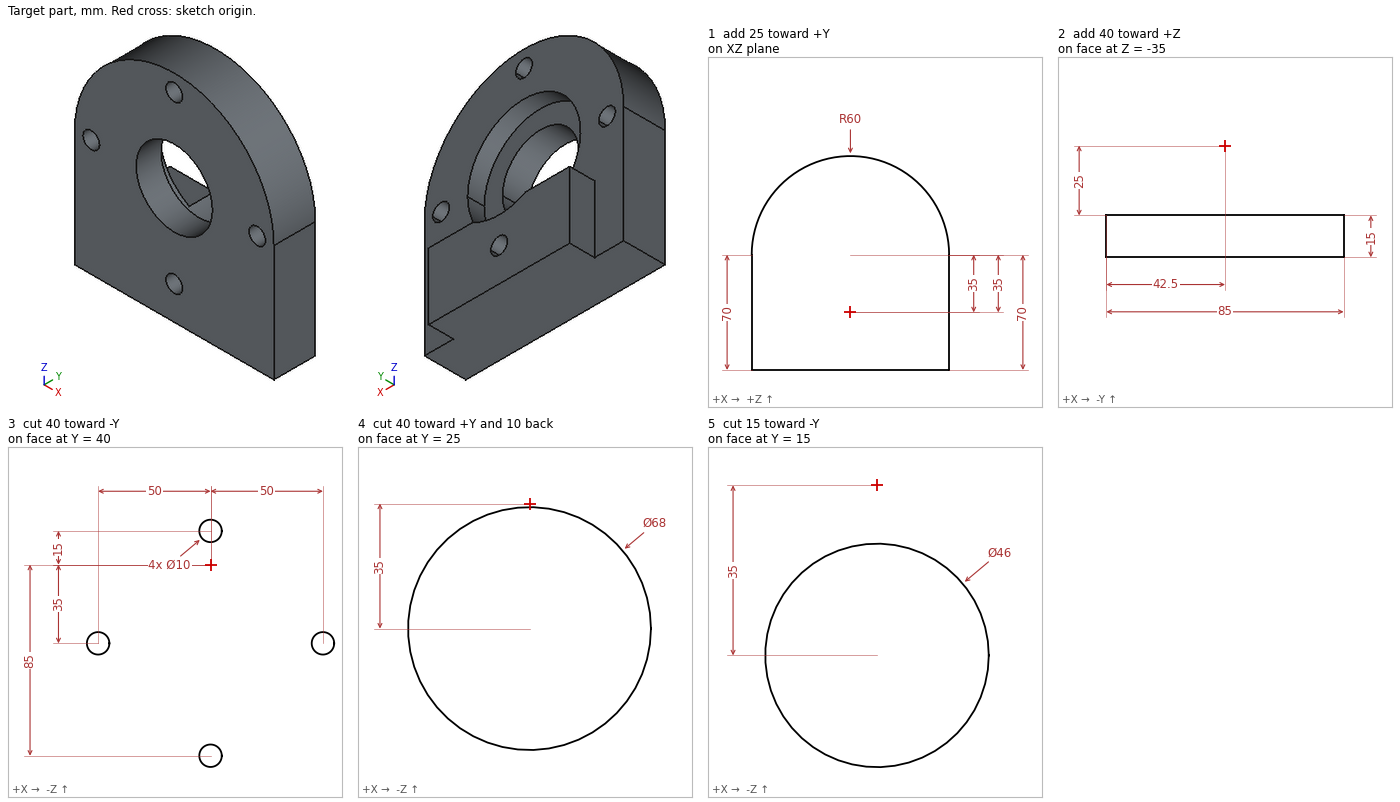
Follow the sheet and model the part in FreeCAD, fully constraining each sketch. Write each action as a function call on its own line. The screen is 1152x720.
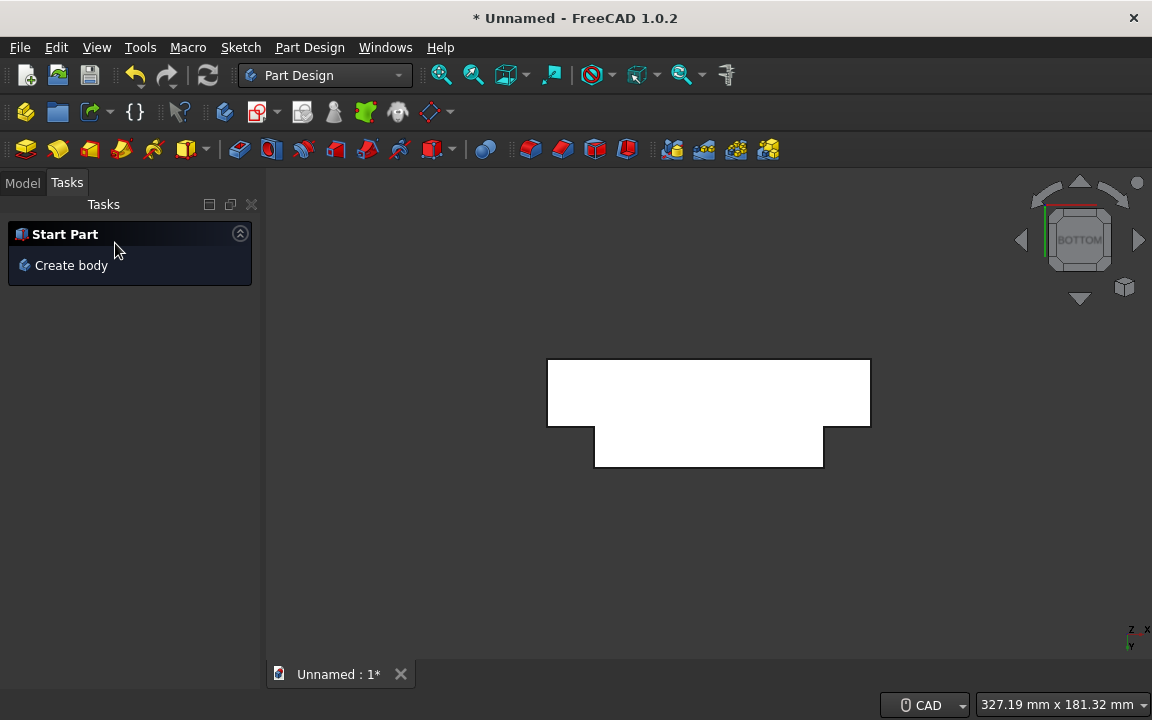
key(4)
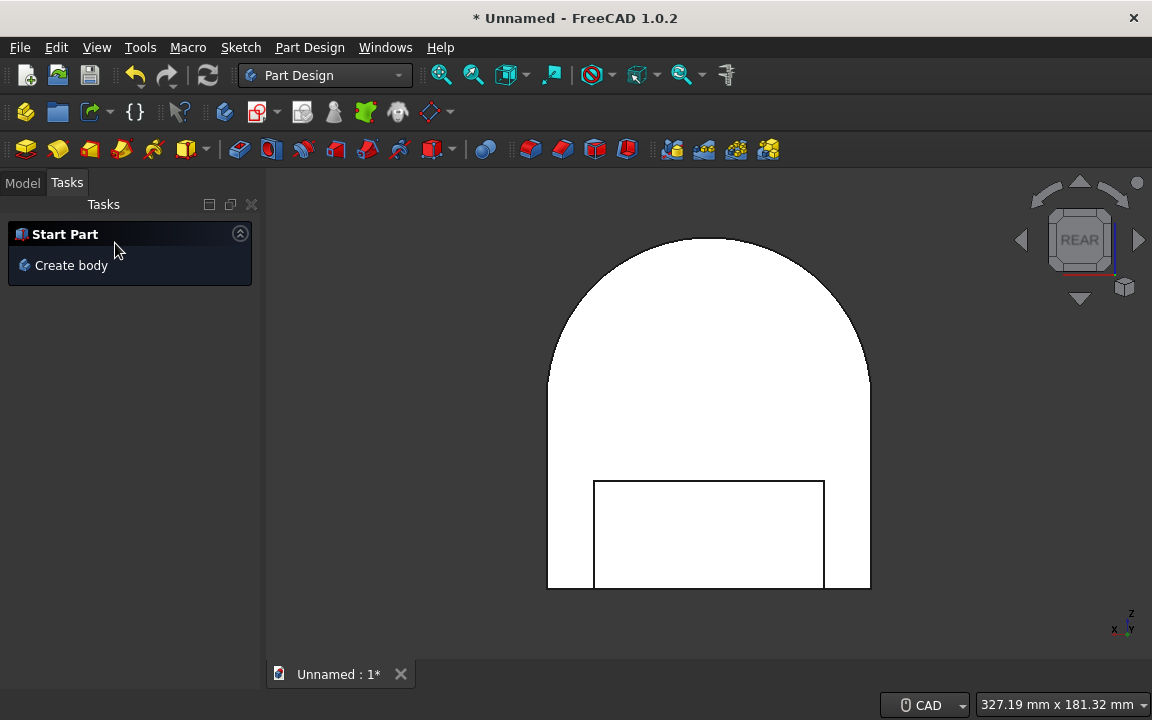
click(676, 534)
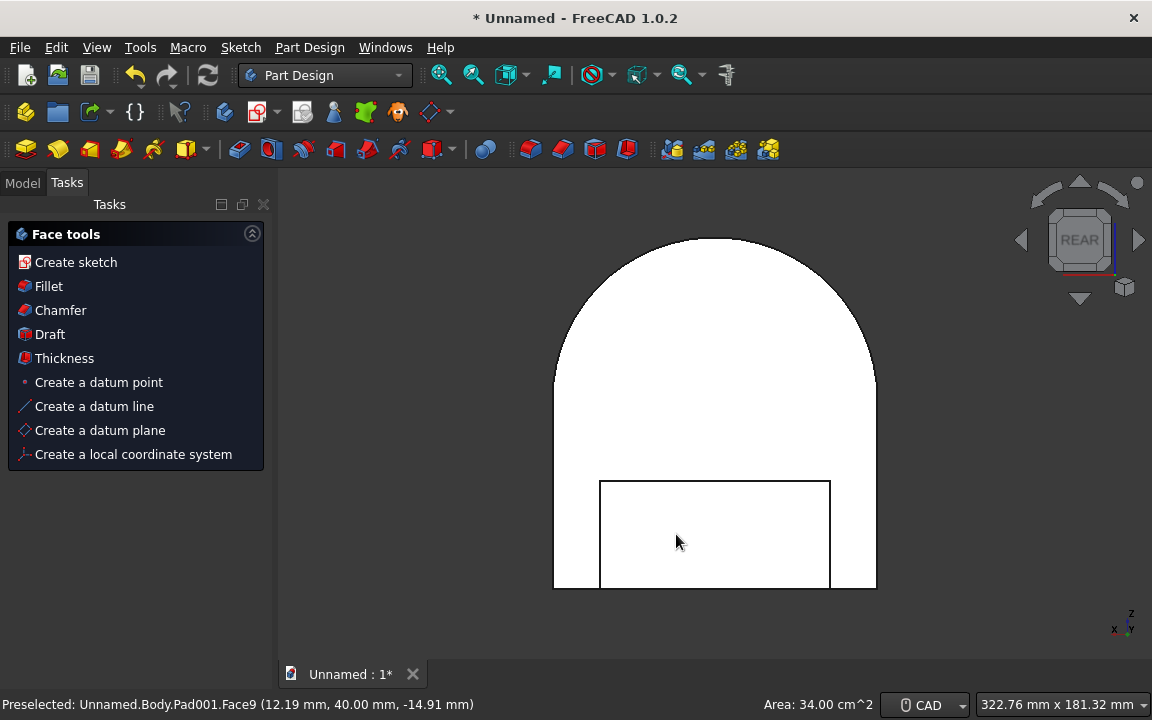
click(258, 112)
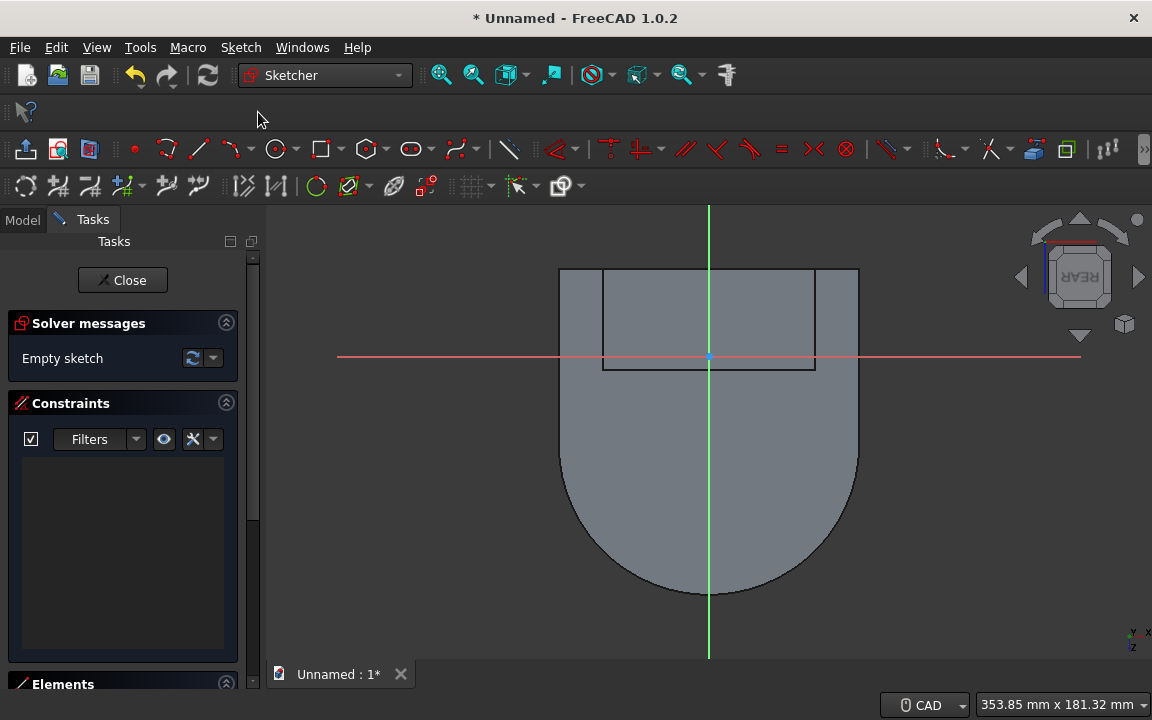
key(g)
key(c)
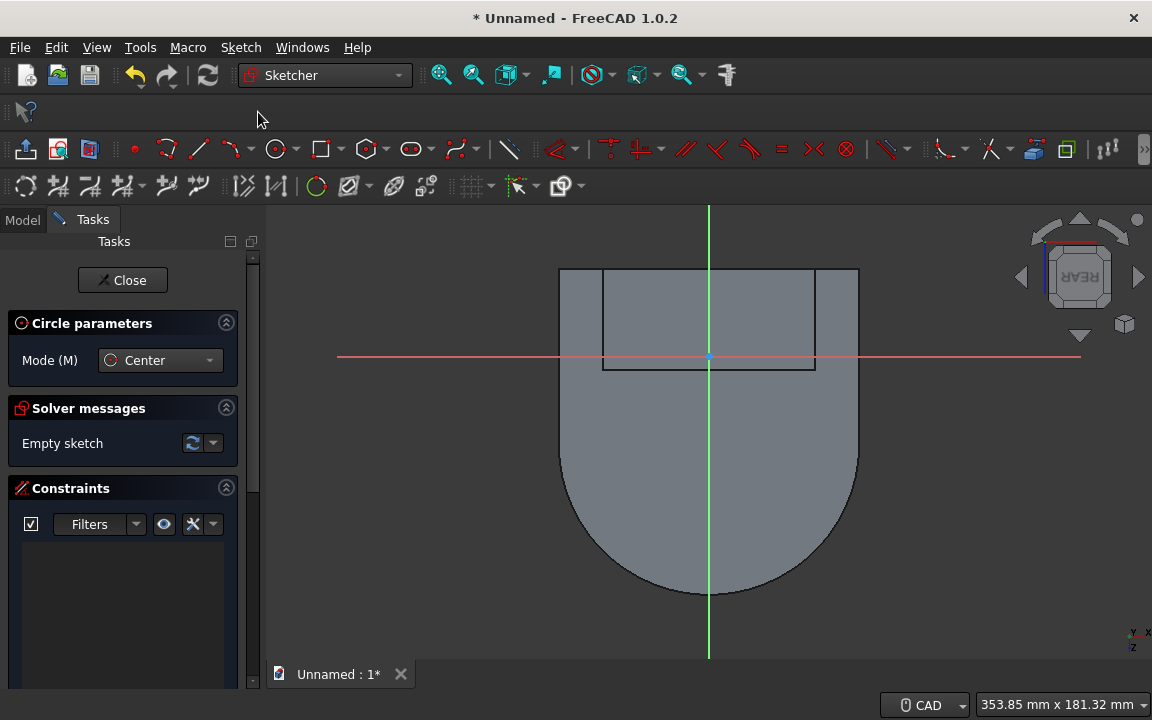
scroll(709, 319, up, 3)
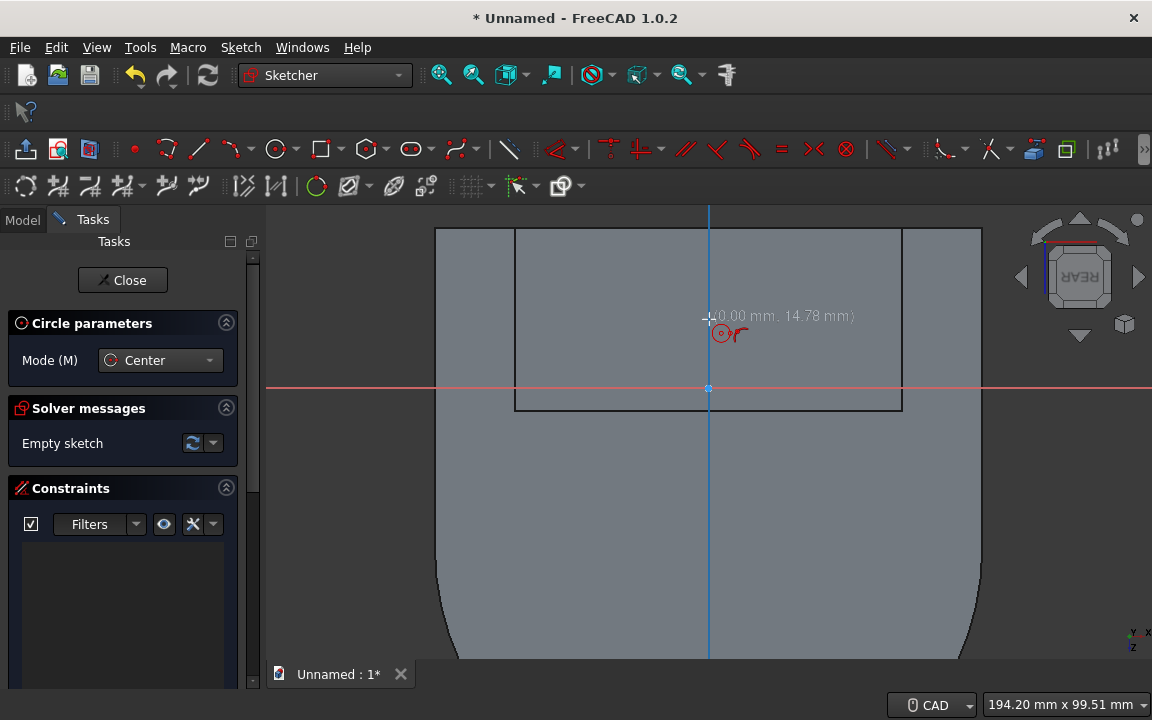
click(709, 320)
move(725, 303)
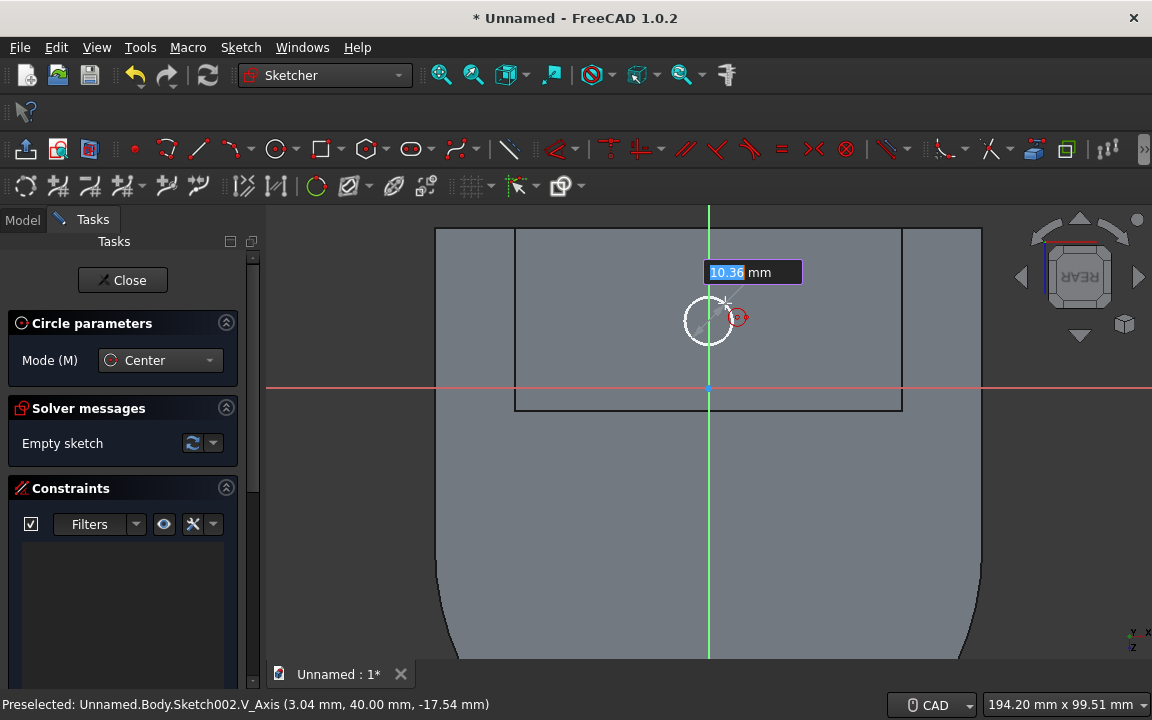
text(10)
key(Return)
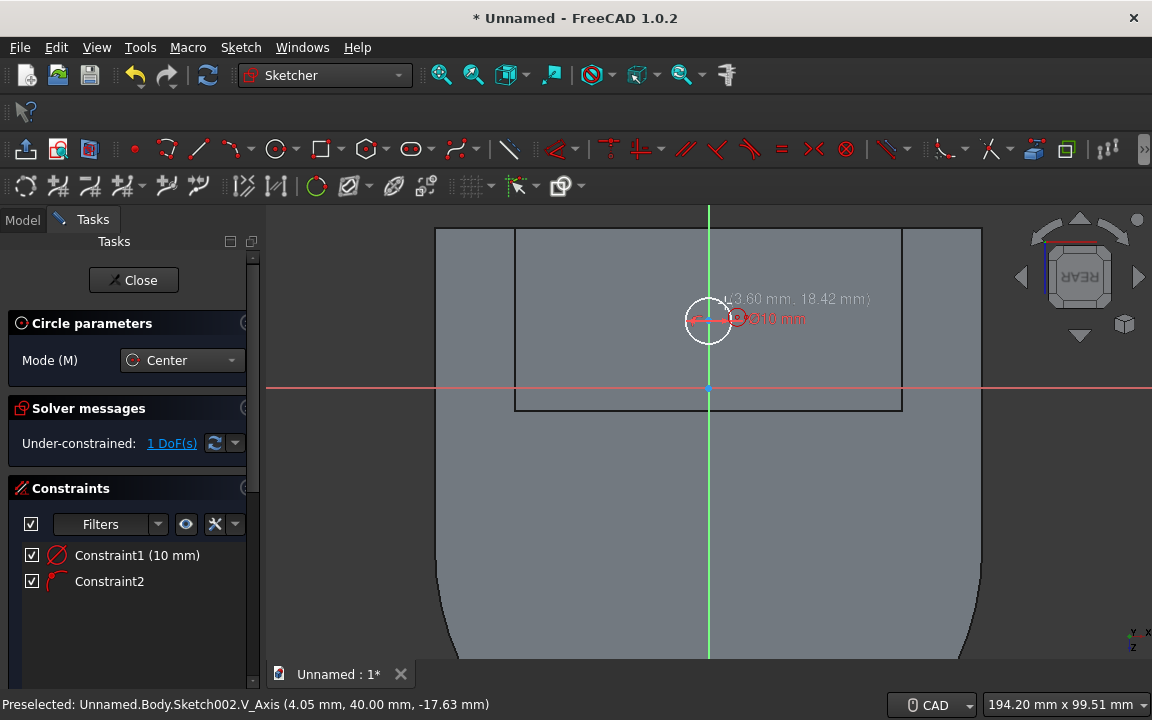
click(480, 548)
move(497, 532)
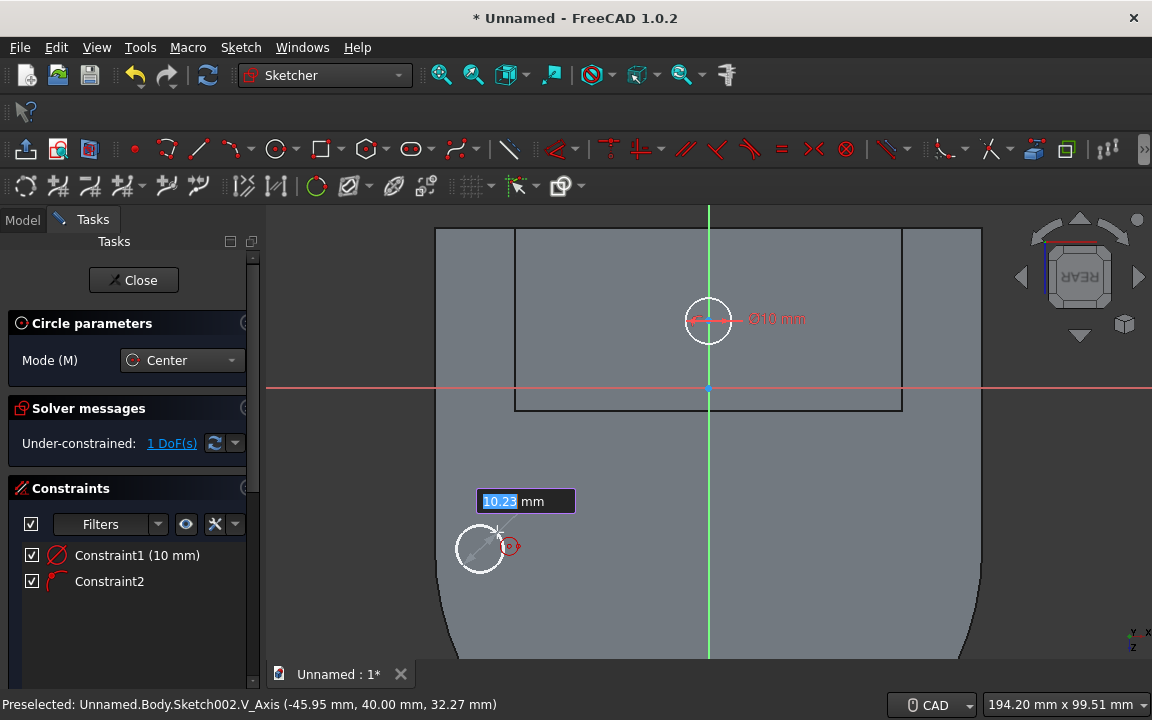
text(10)
key(Return)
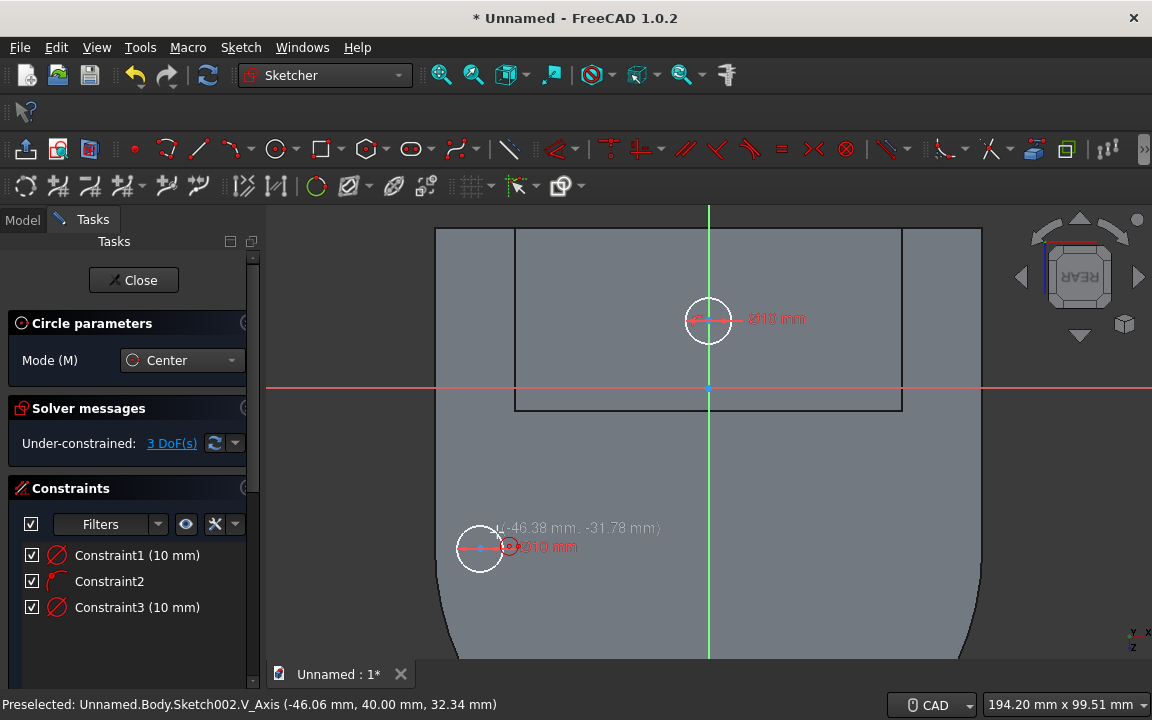
click(937, 548)
move(953, 532)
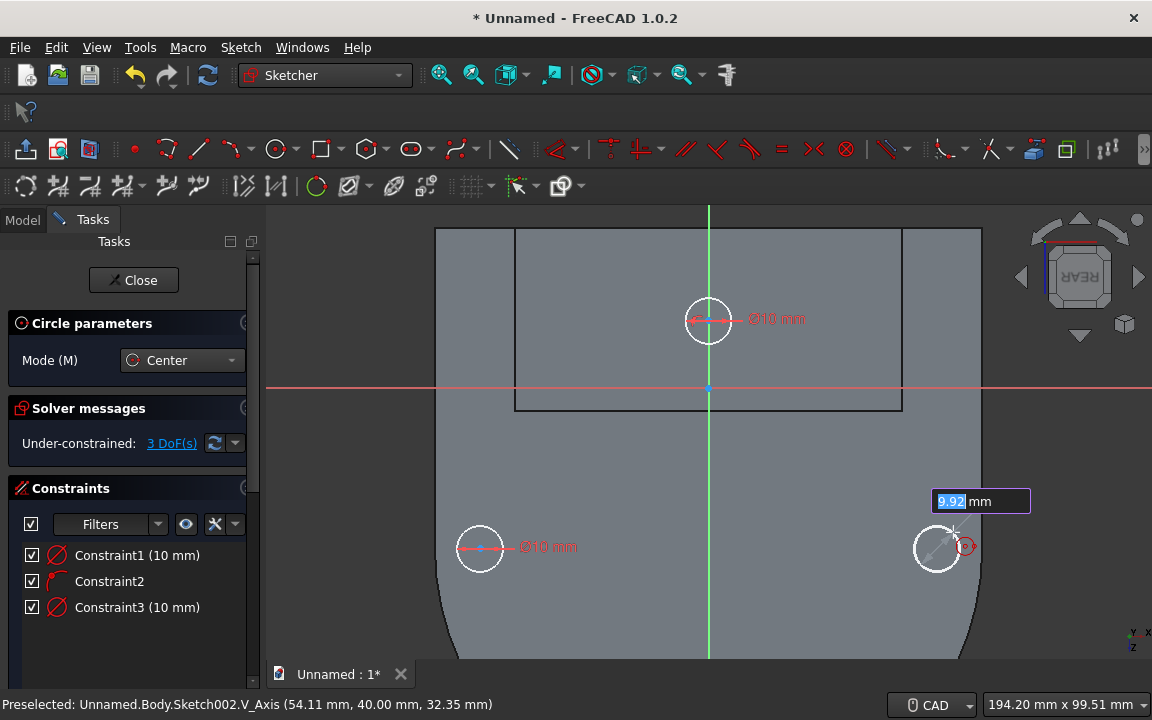
text(10)
key(Return)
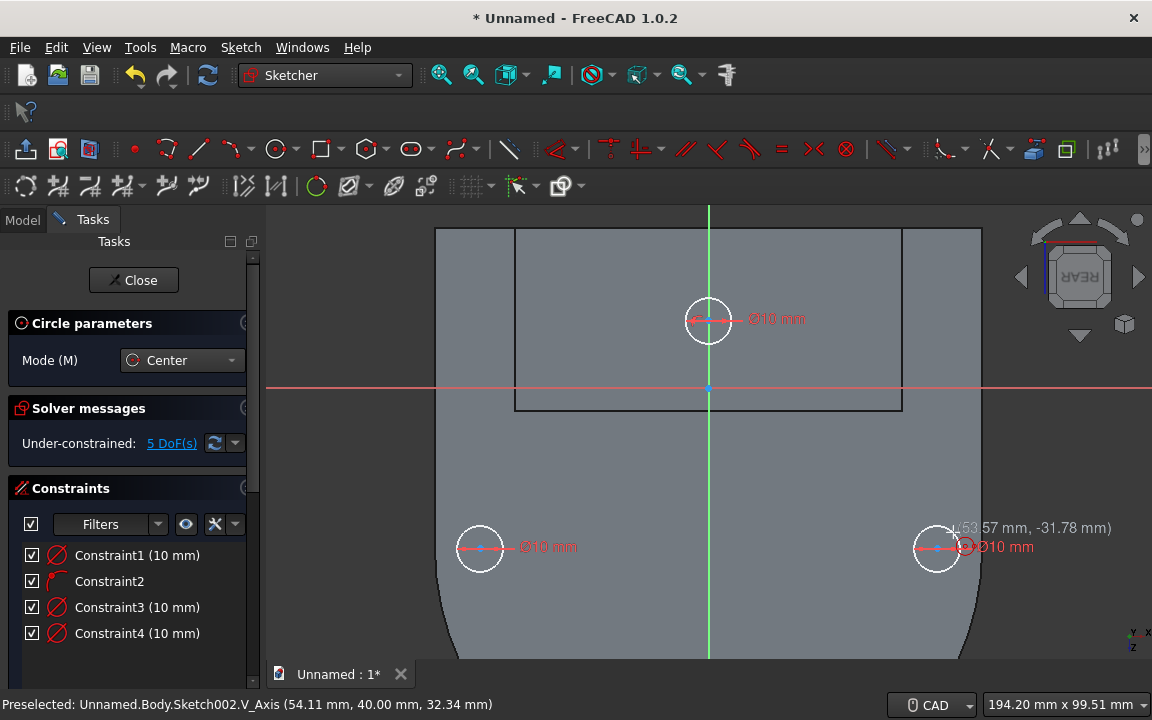
scroll(558, 291, down, 3)